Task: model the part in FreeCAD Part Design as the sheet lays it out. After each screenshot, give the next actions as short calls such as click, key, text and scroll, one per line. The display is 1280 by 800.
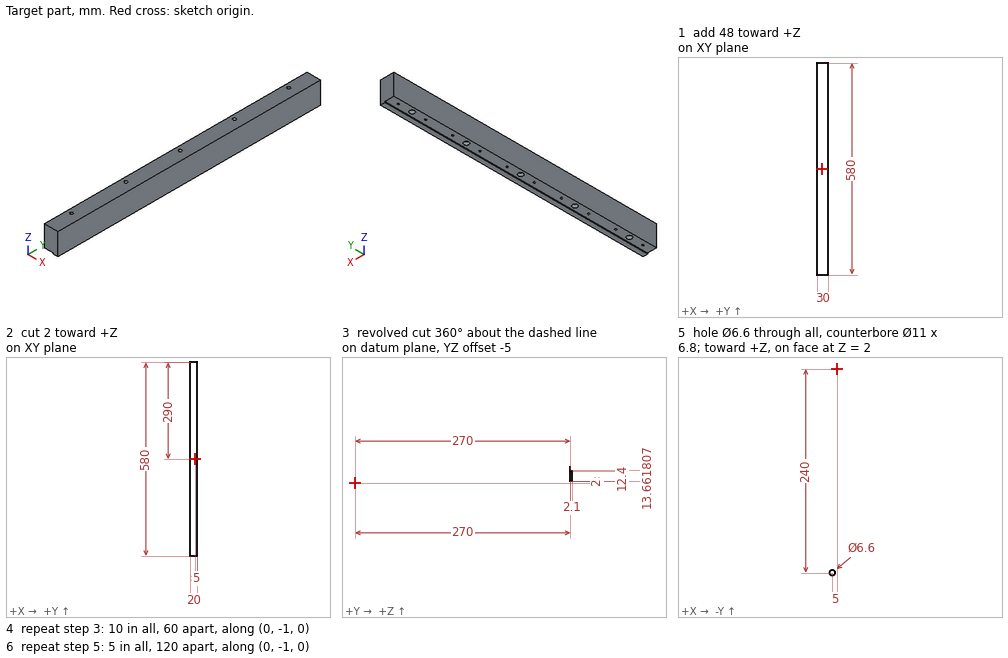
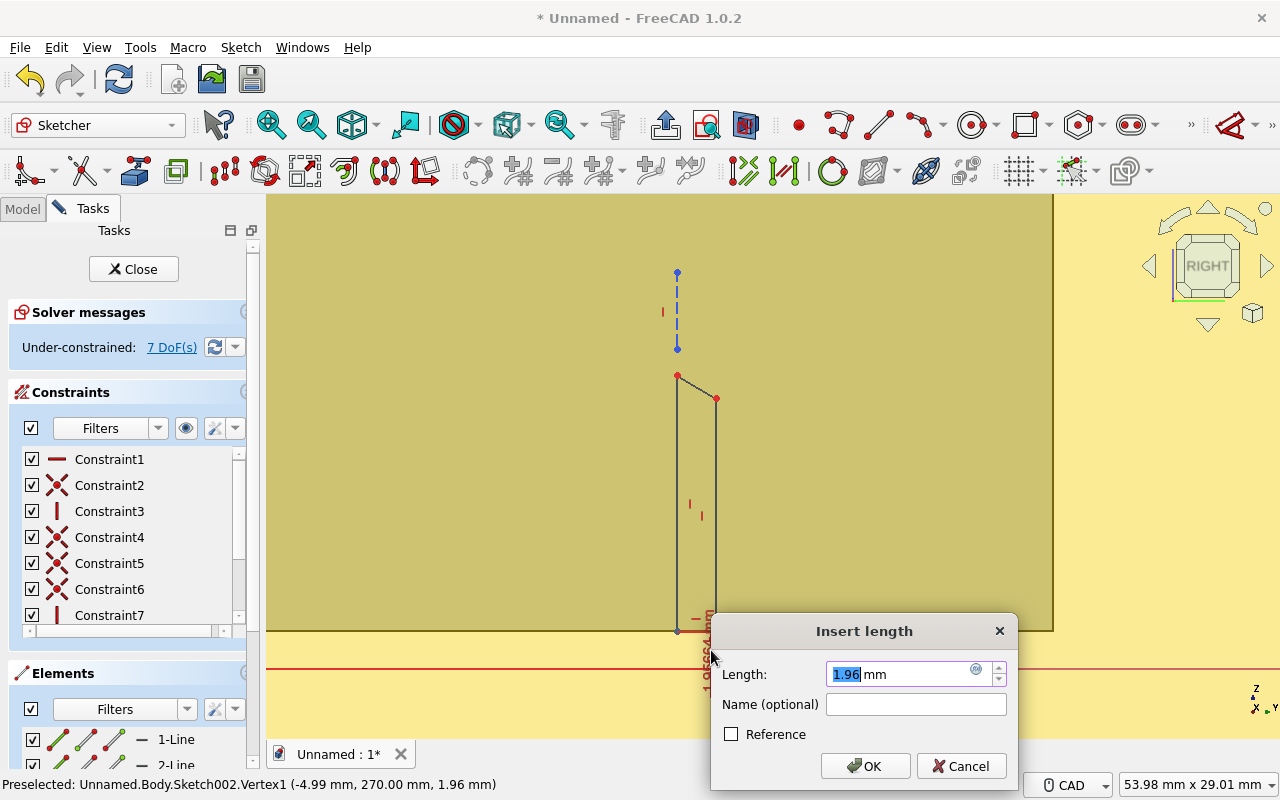
text(2)
key(Return)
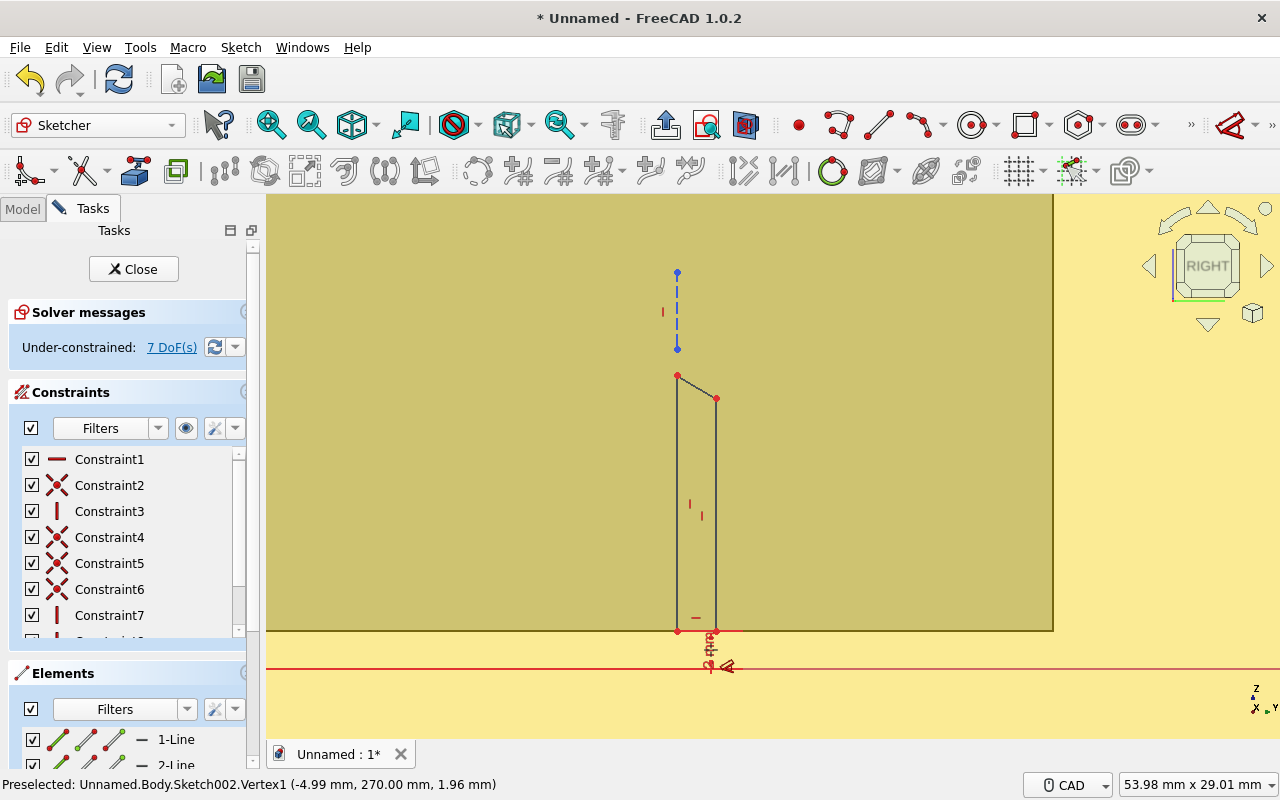
click(689, 631)
click(697, 597)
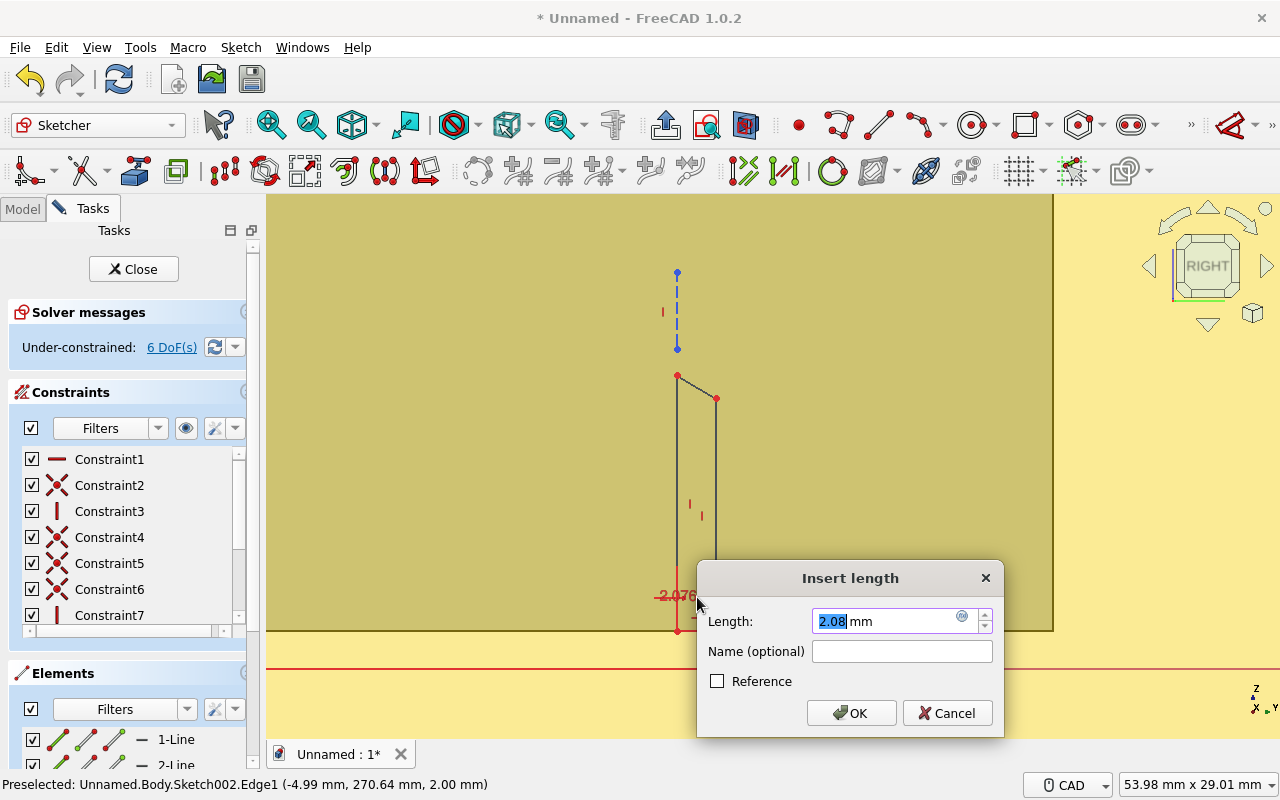
text(2.1)
key(Return)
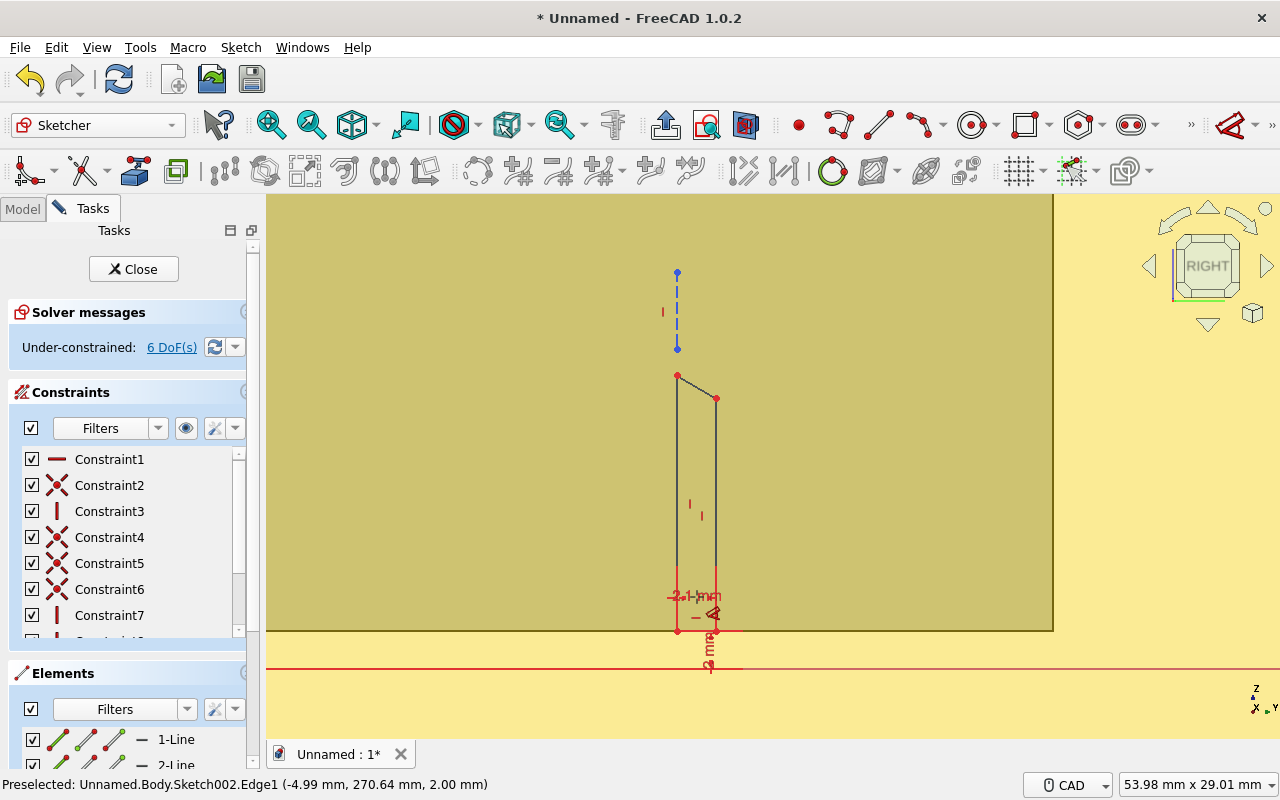
click(716, 562)
click(750, 515)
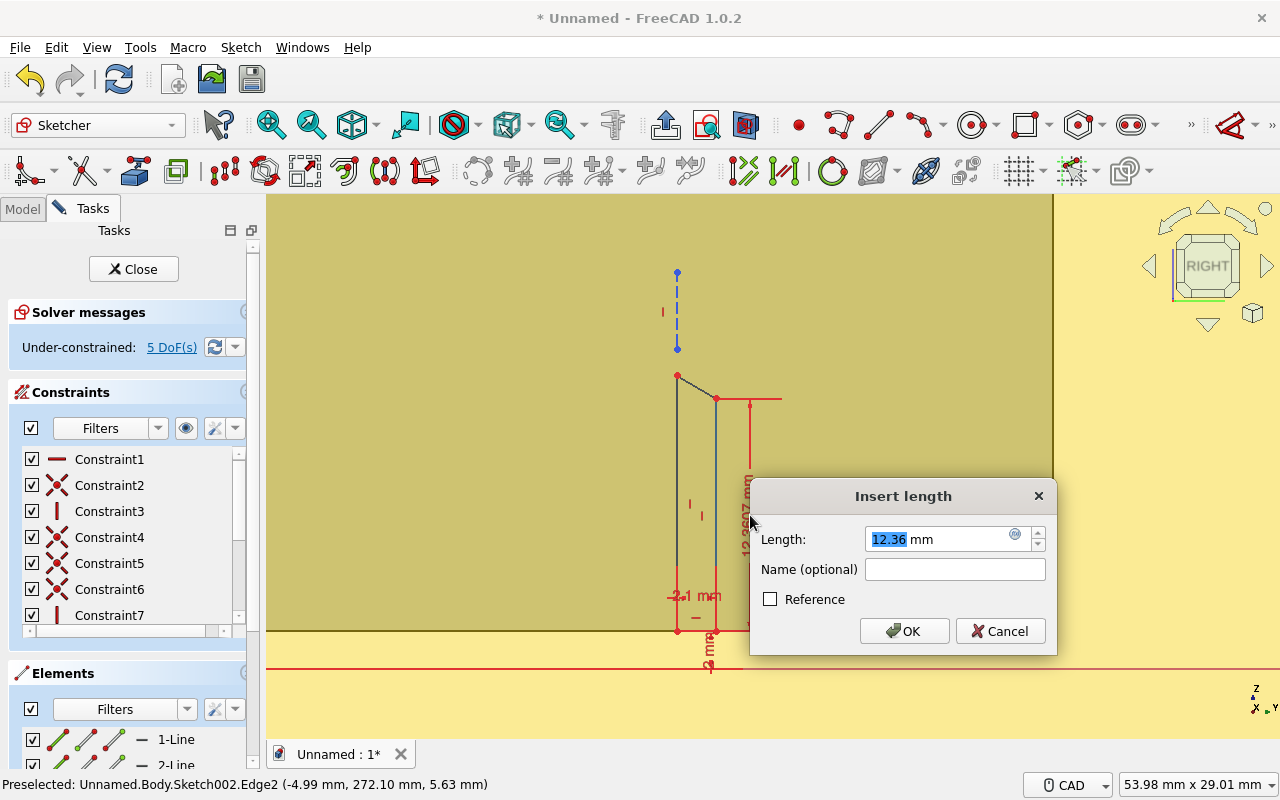
text(12.4)
key(Return)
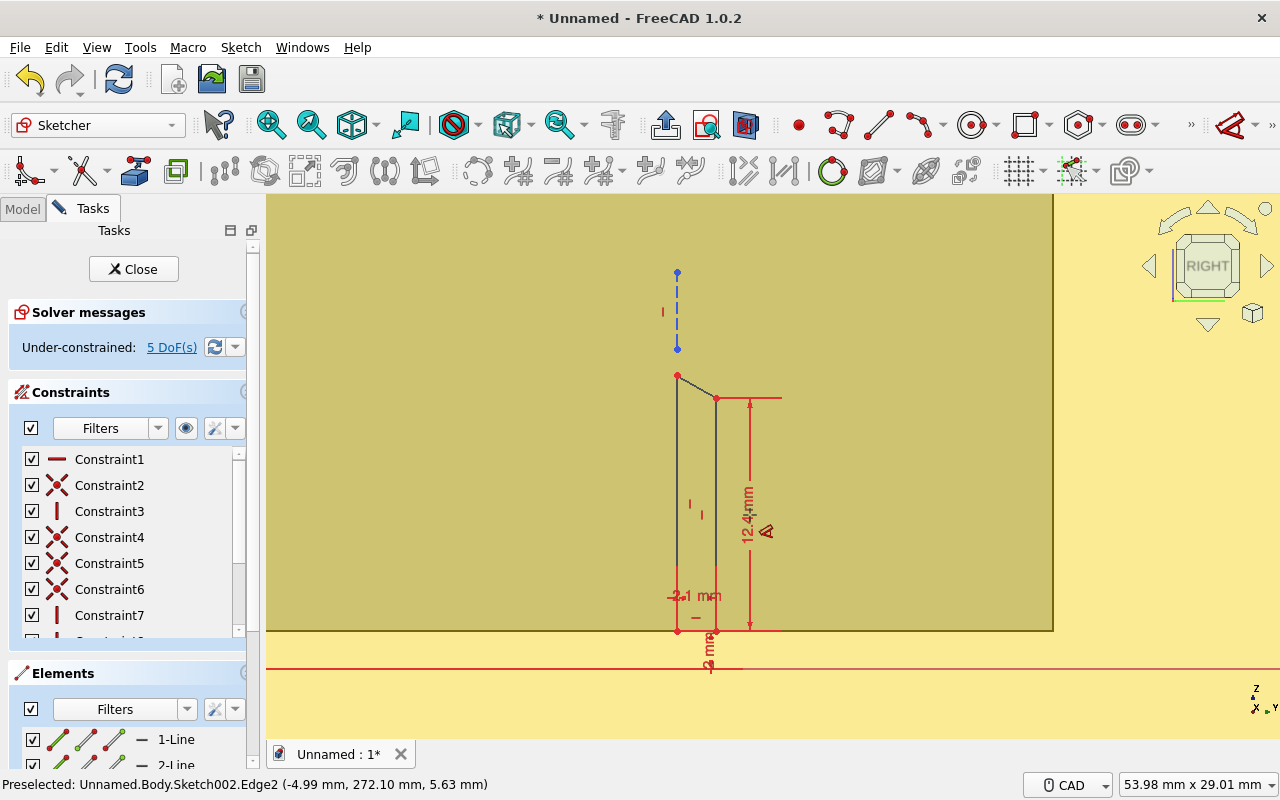
click(677, 631)
click(486, 703)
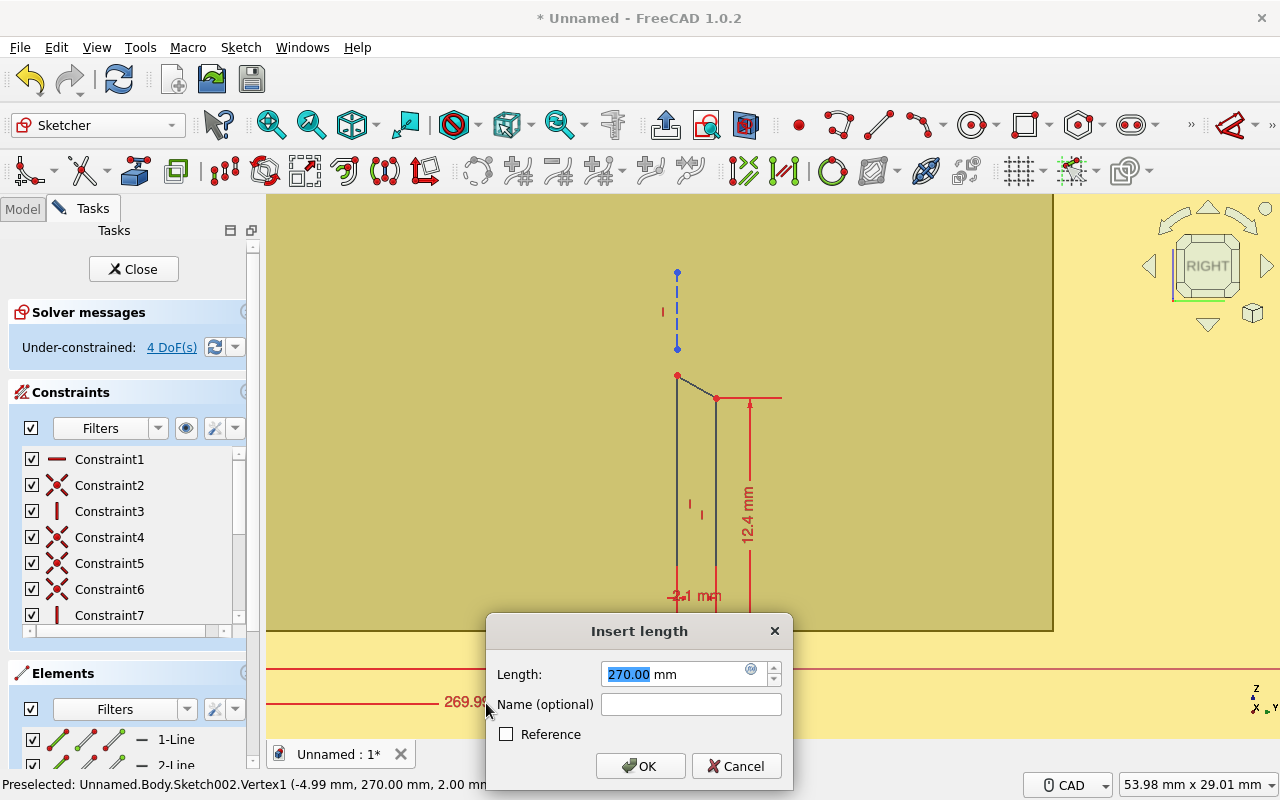
text(270)
key(Return)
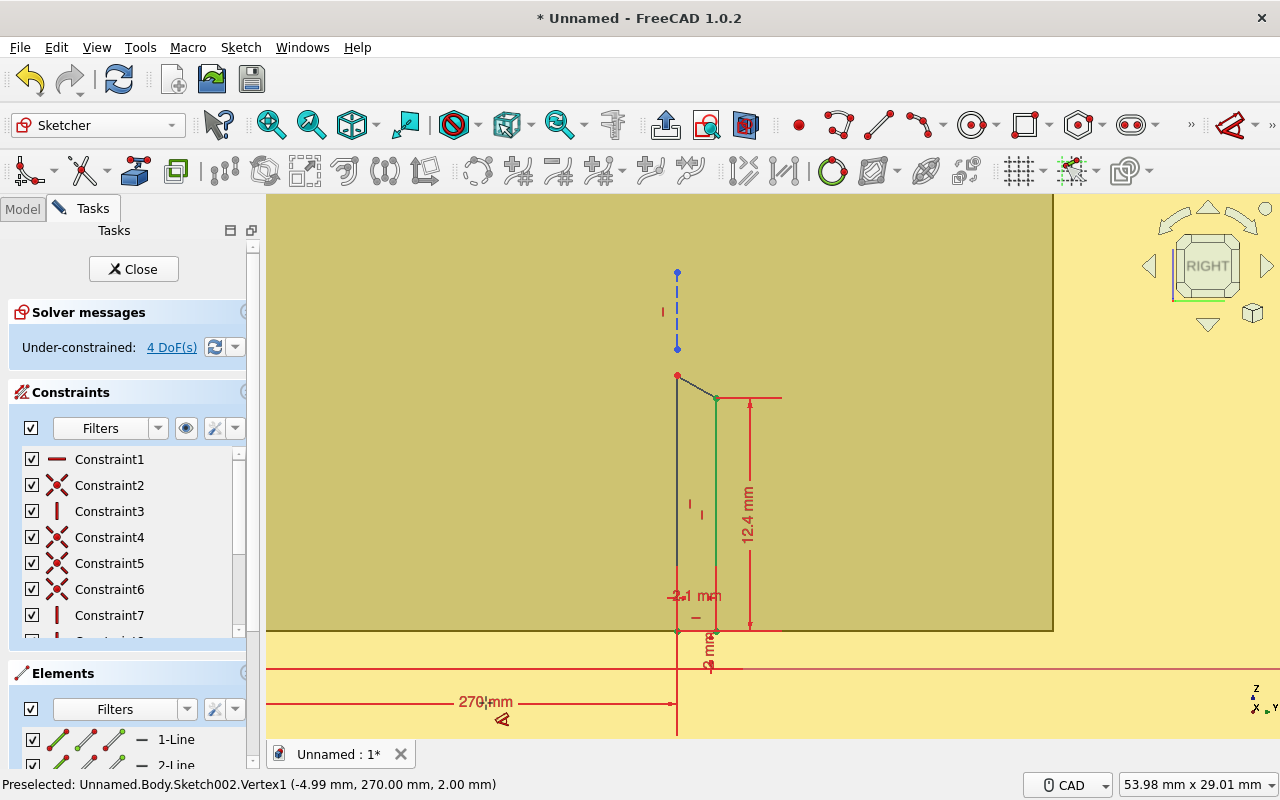
click(677, 350)
click(397, 703)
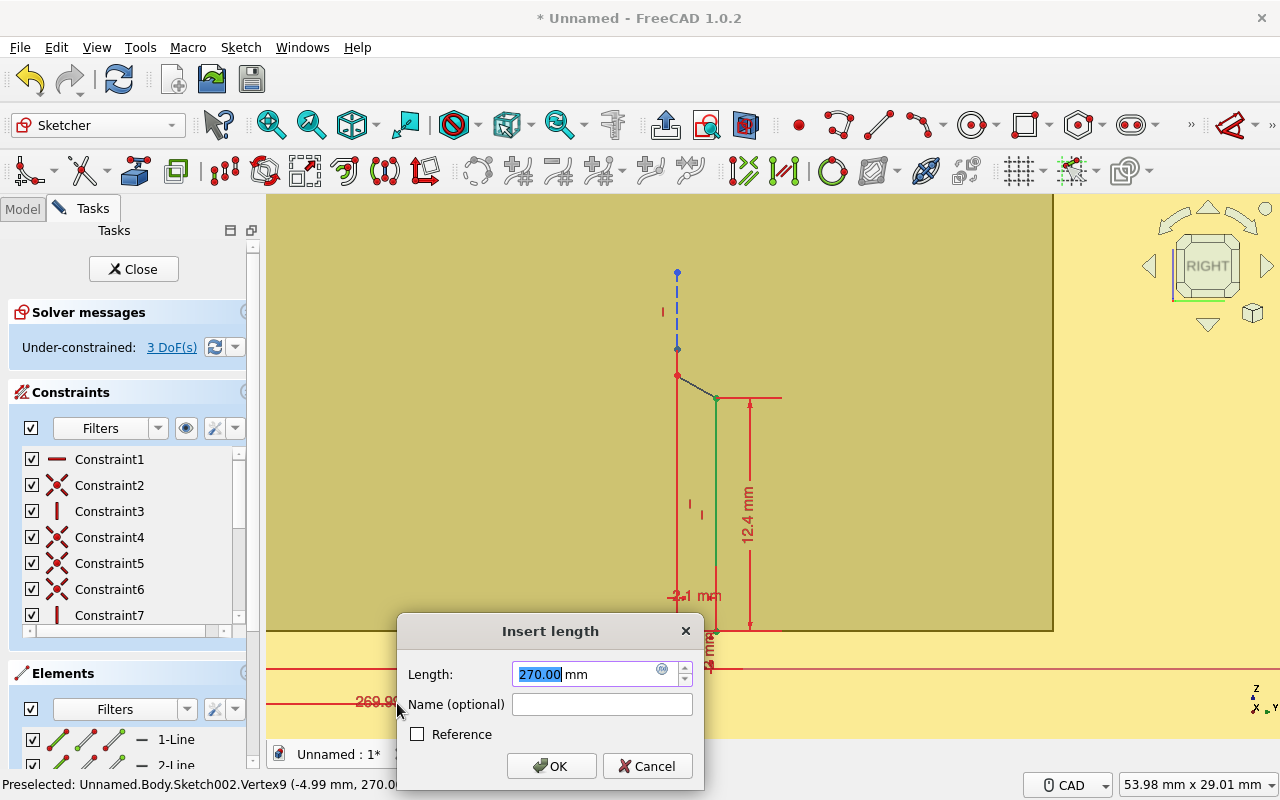
text(270)
key(Return)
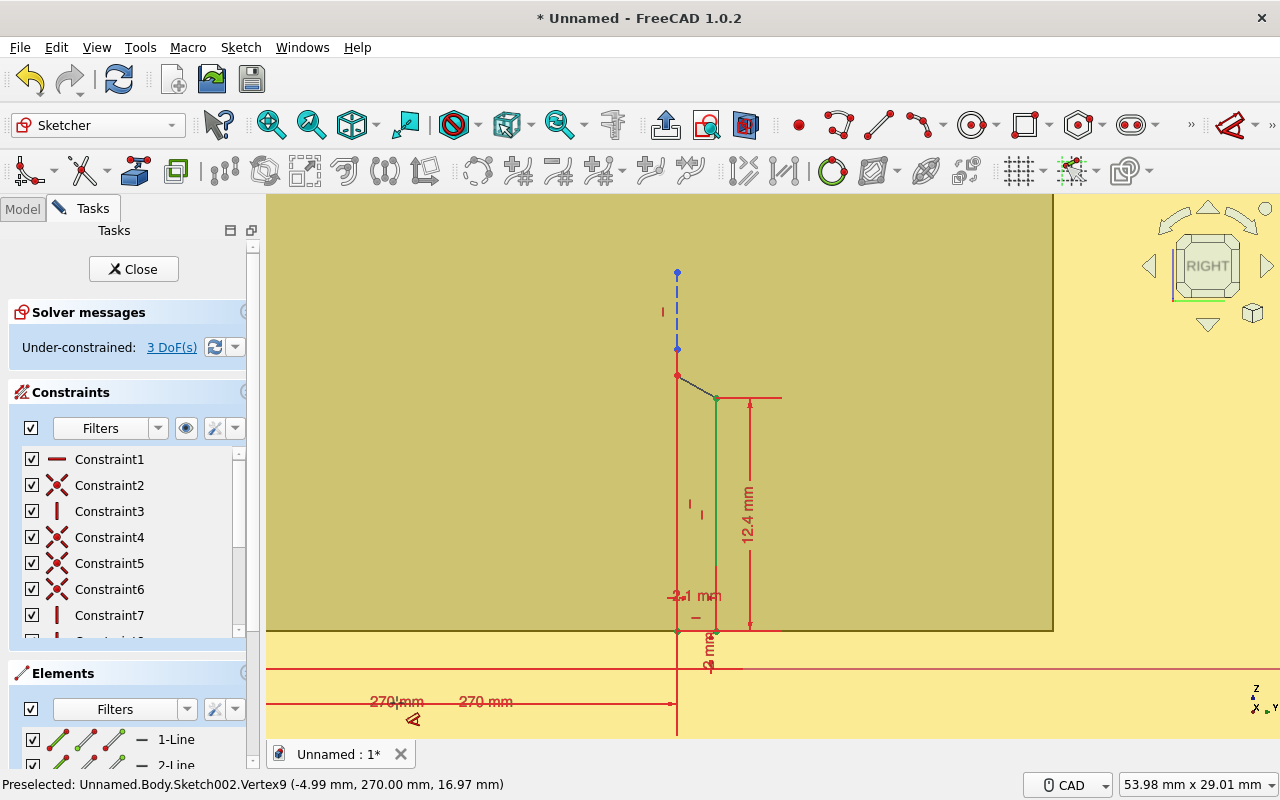
click(677, 453)
click(643, 504)